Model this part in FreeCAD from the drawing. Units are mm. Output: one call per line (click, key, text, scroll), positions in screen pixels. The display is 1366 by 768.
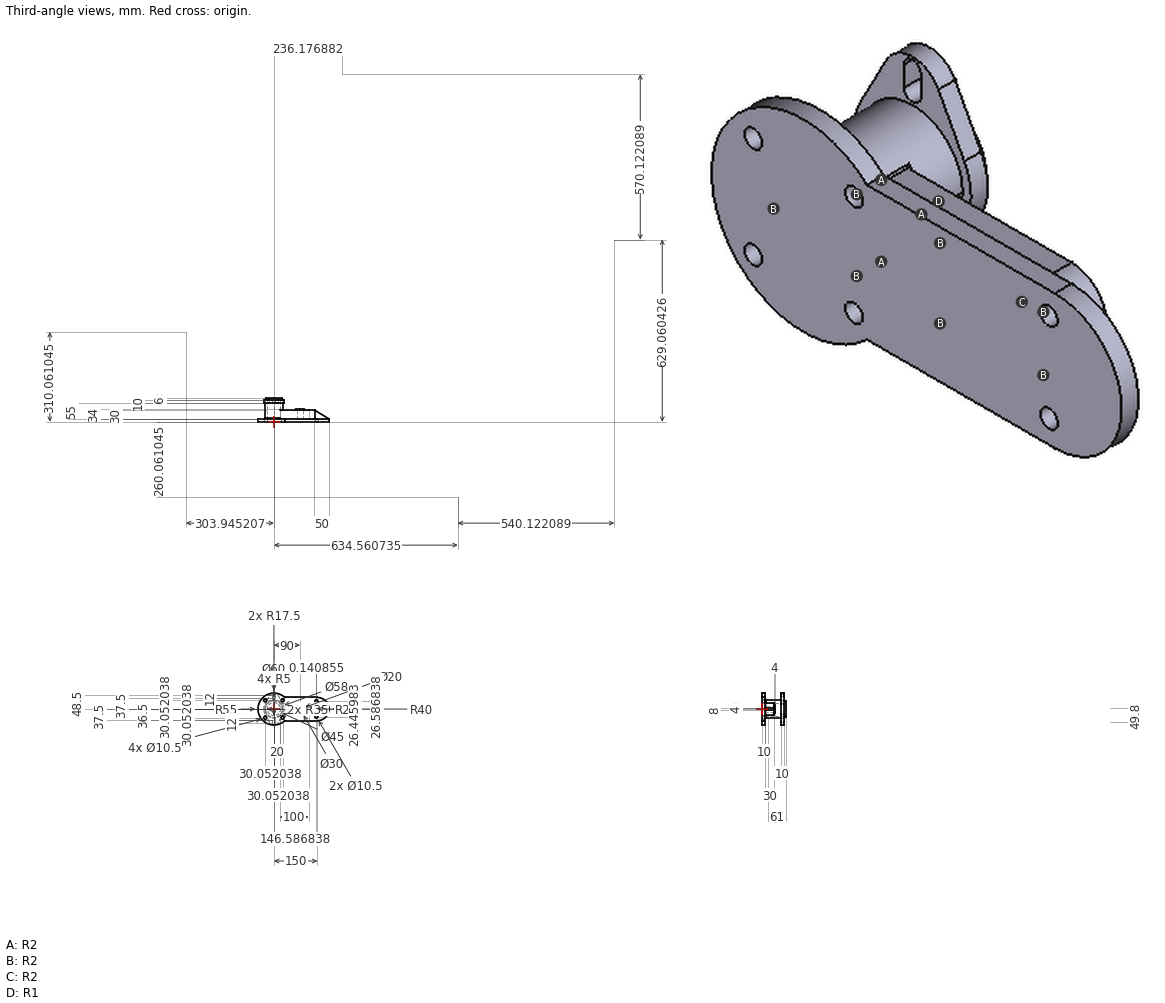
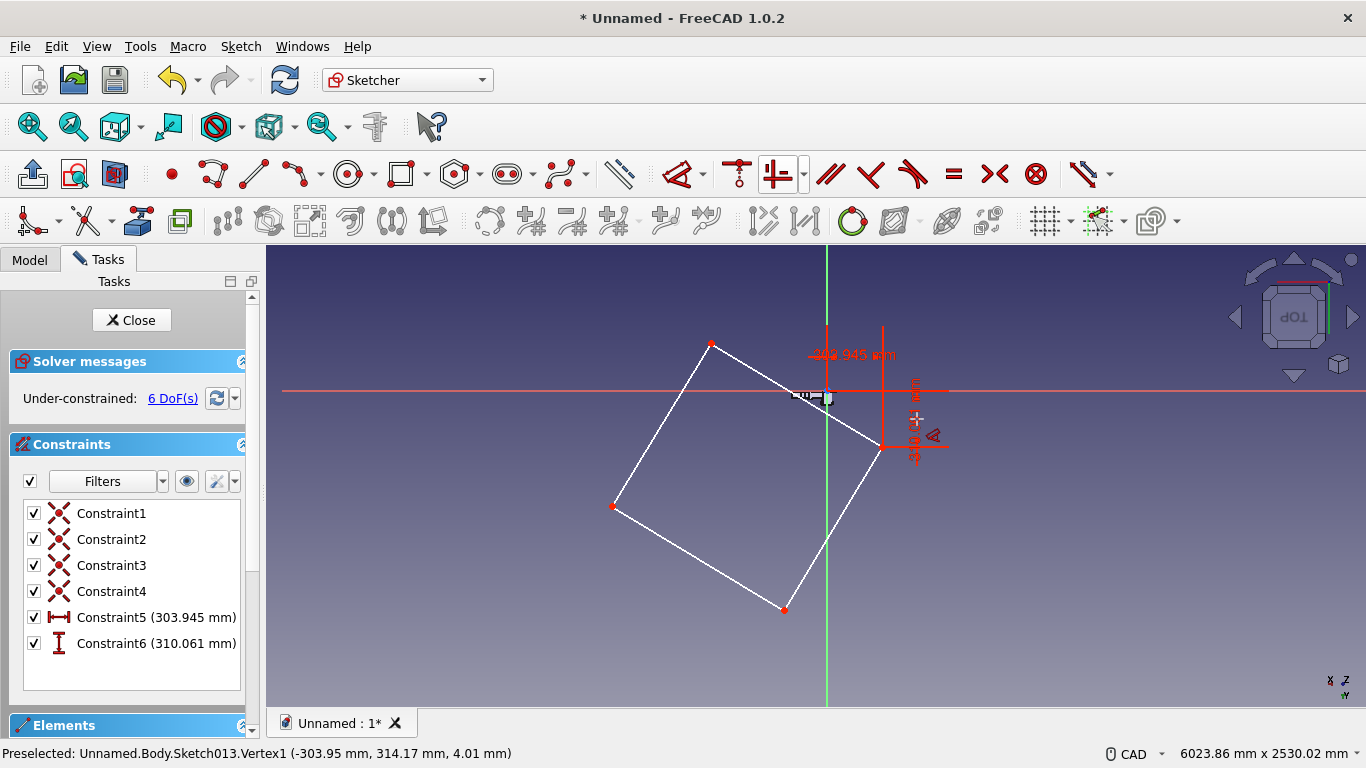
click(711, 344)
click(769, 310)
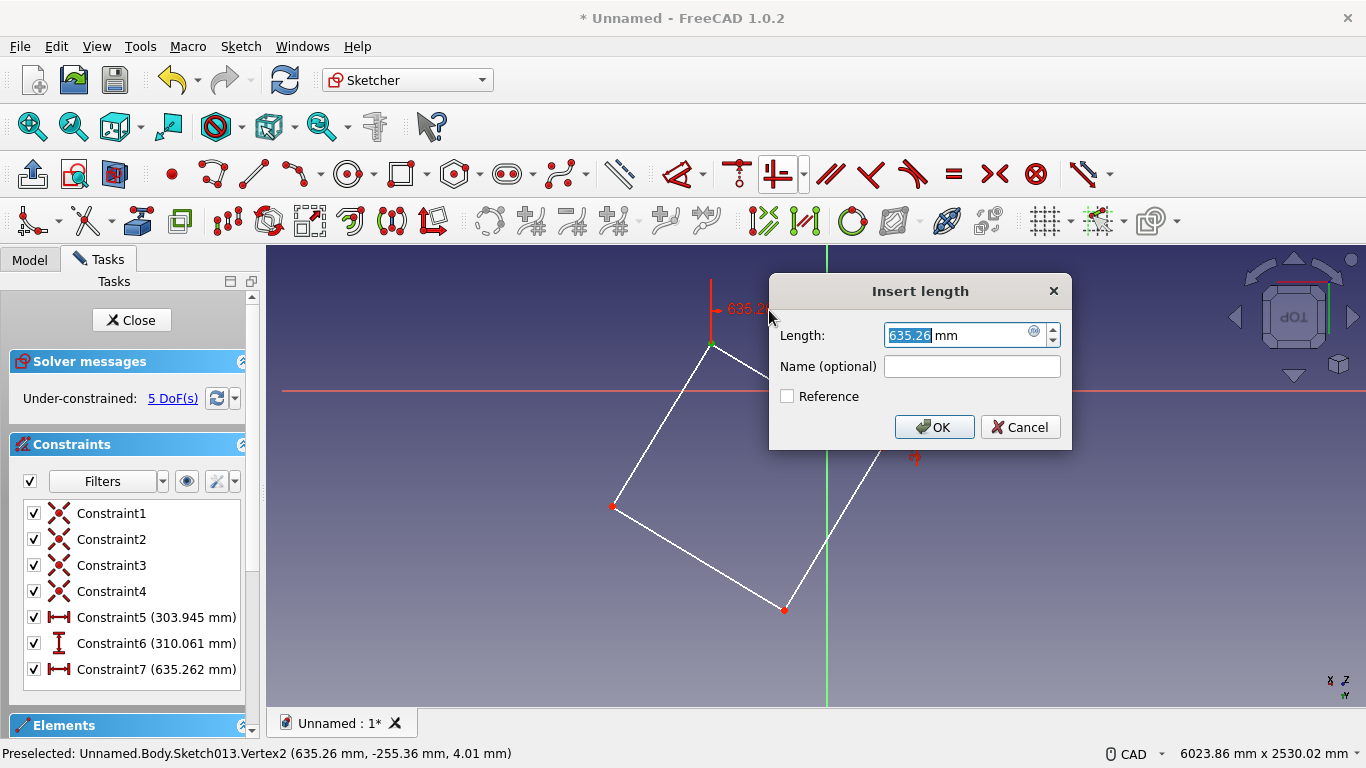
text(634.560735)
key(Return)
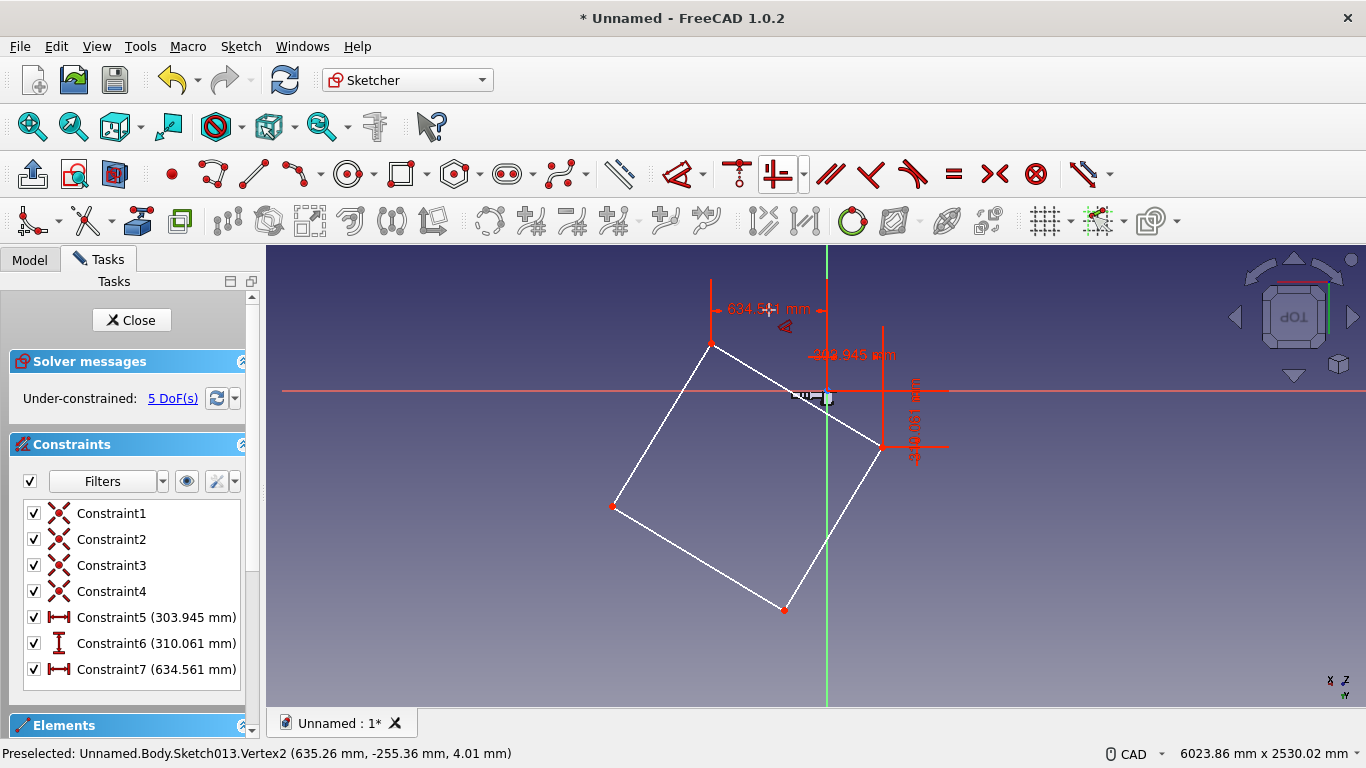
click(711, 344)
click(677, 367)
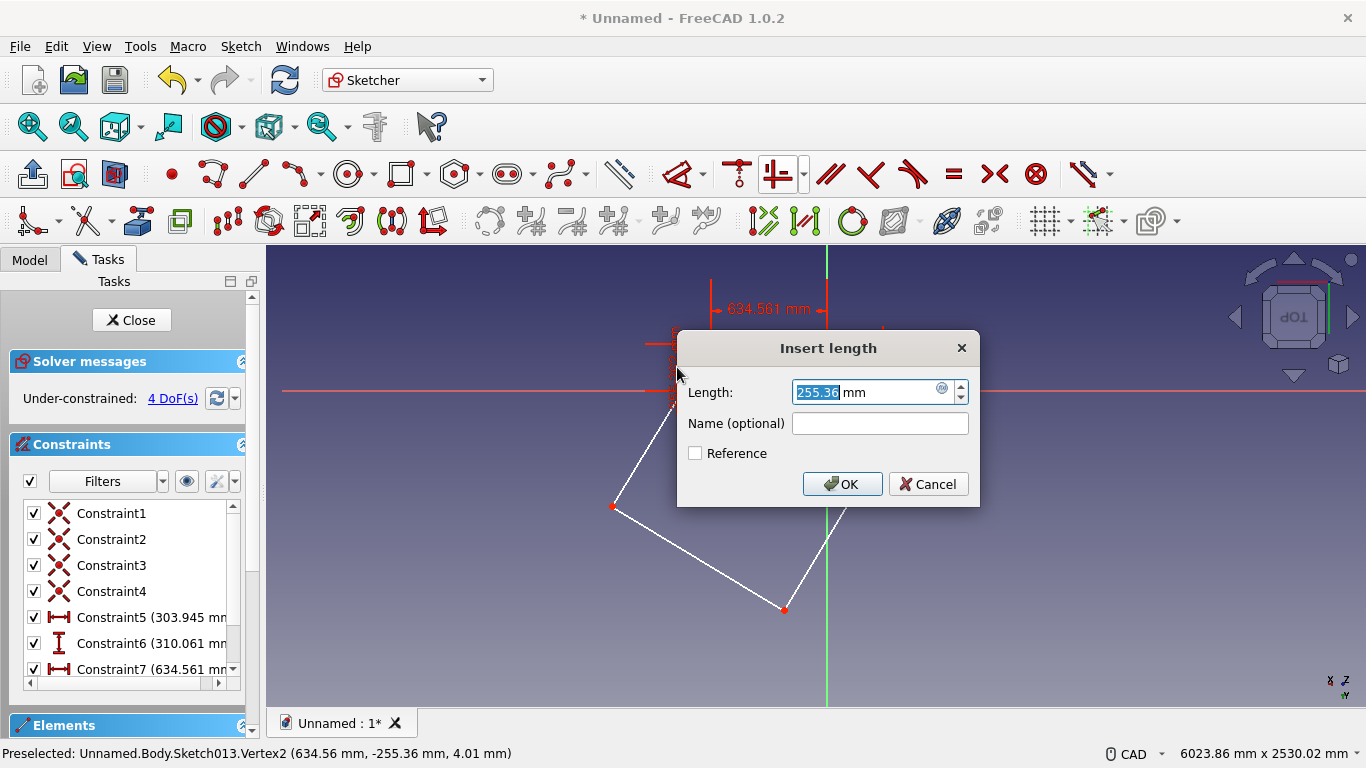
text(260.061045)
key(Return)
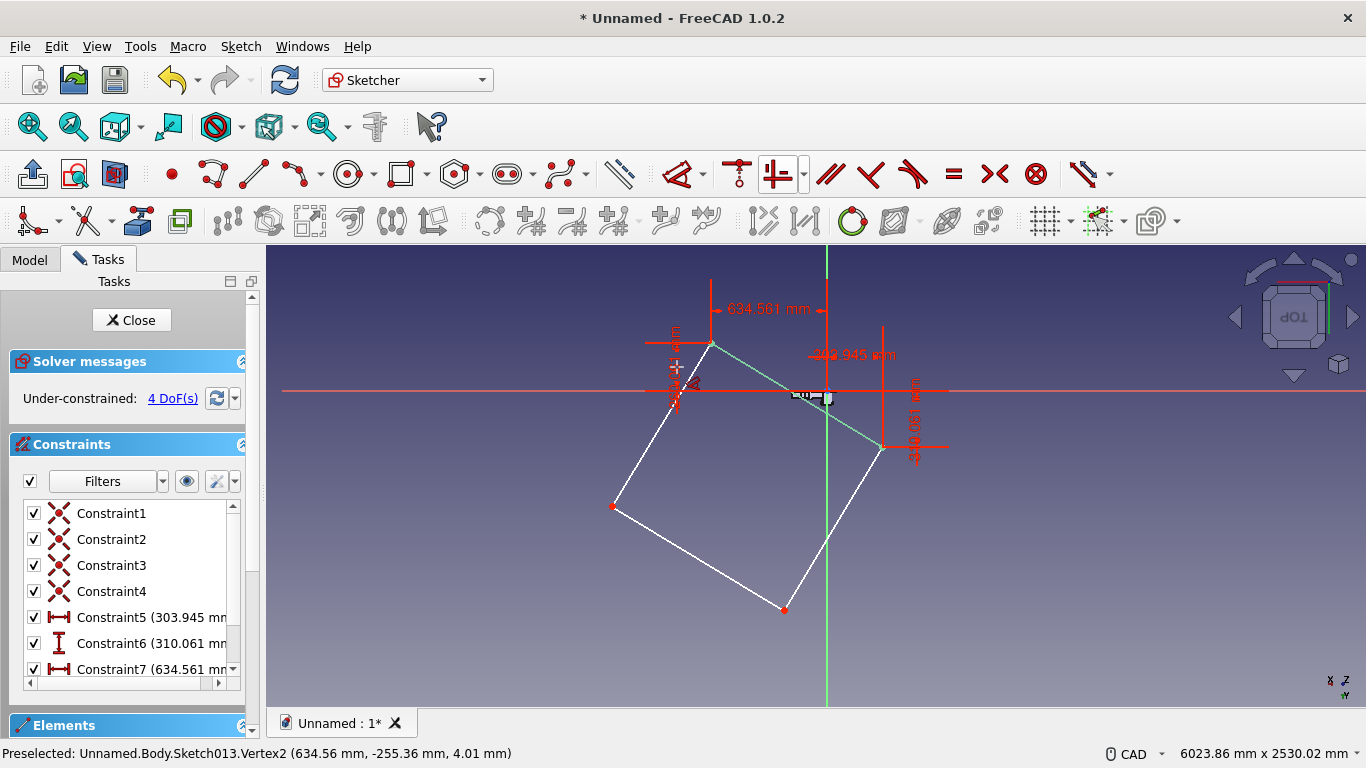
click(612, 507)
click(578, 449)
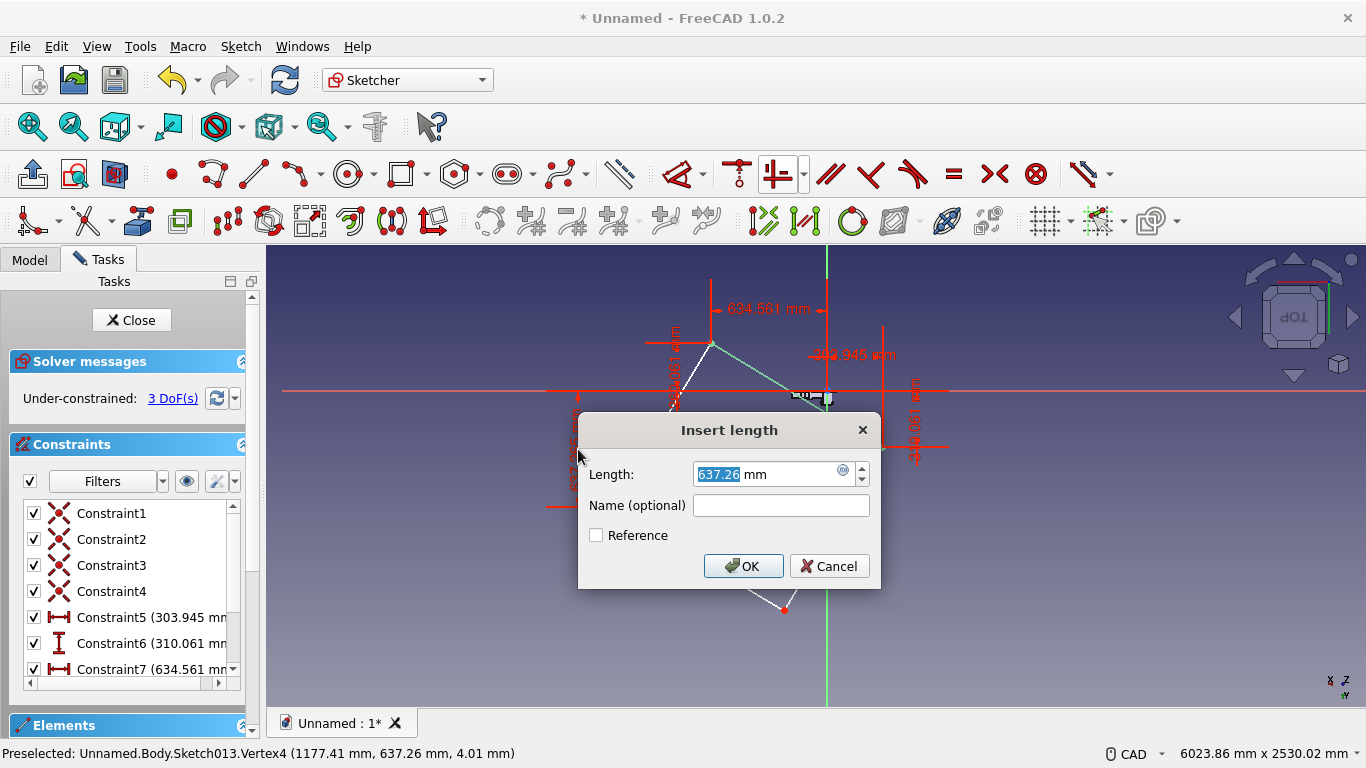
text(629.060426)
key(Return)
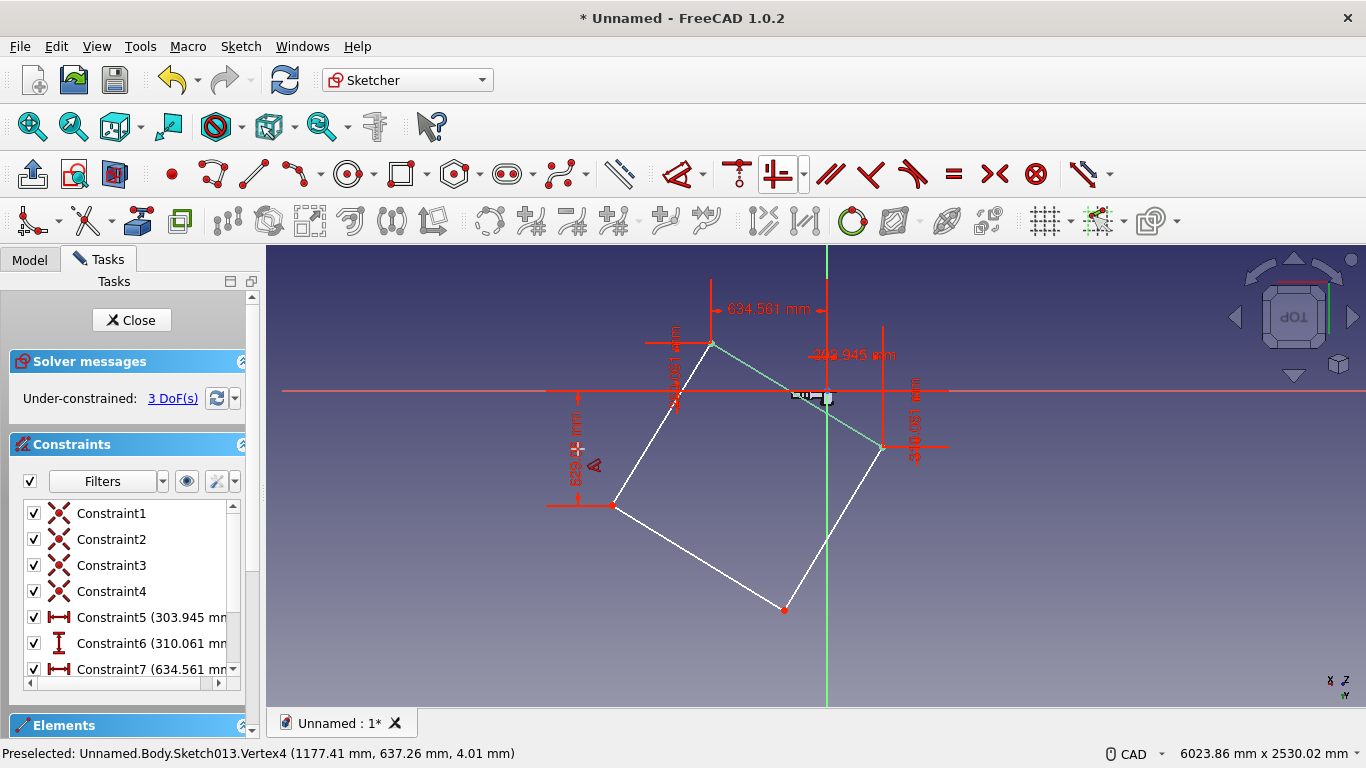
click(784, 611)
click(806, 645)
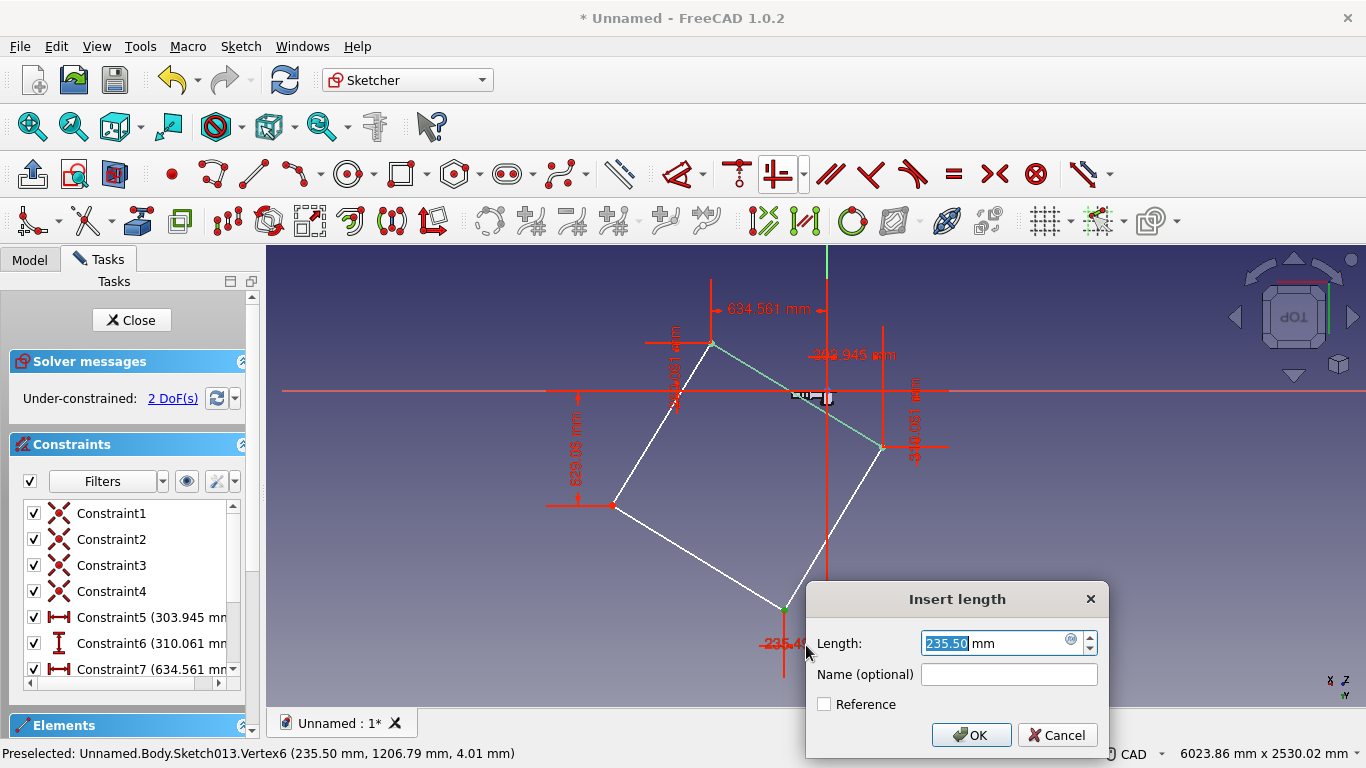
text(236.176882)
key(Return)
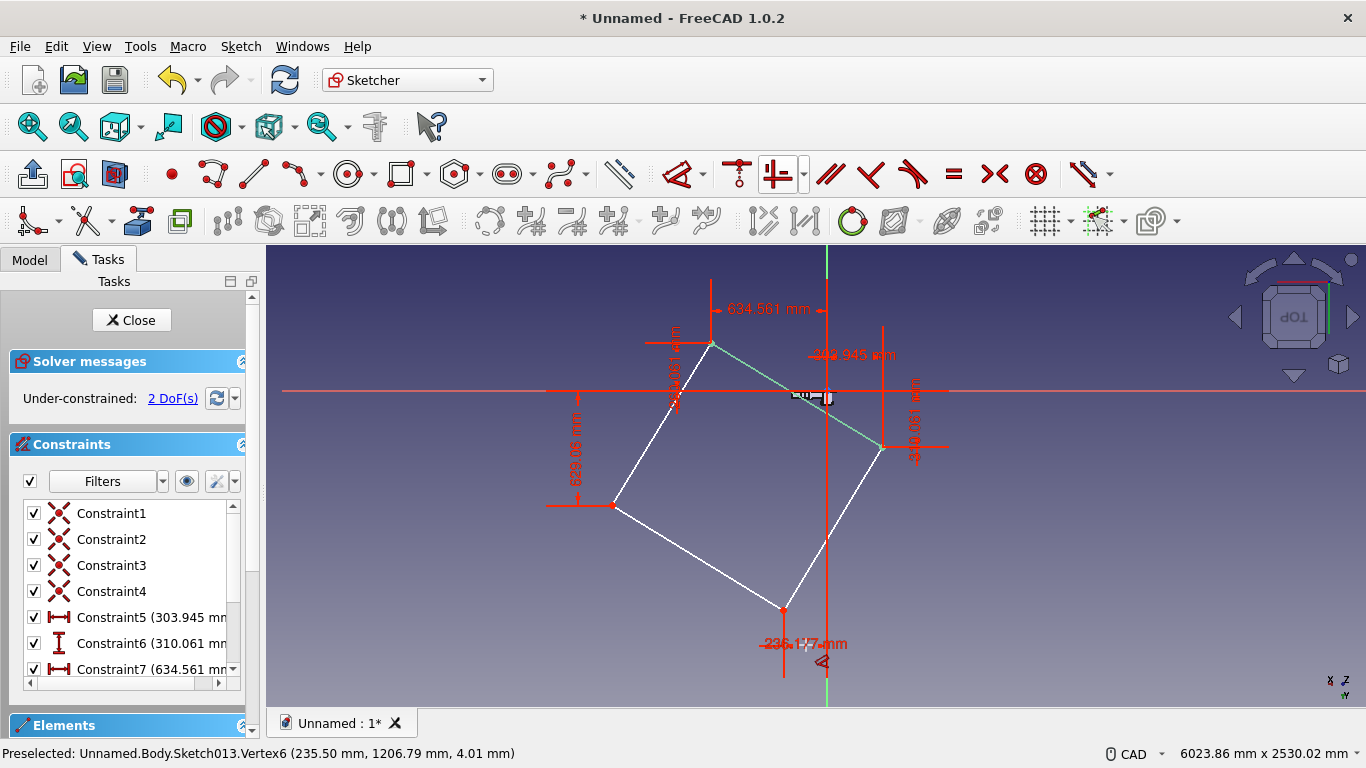
click(681, 392)
click(662, 309)